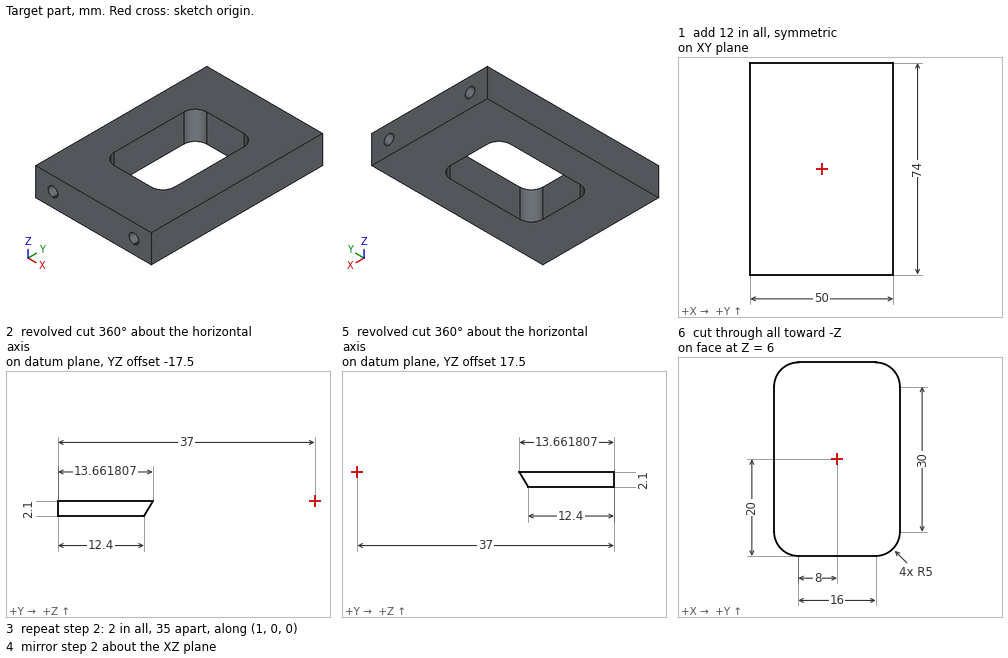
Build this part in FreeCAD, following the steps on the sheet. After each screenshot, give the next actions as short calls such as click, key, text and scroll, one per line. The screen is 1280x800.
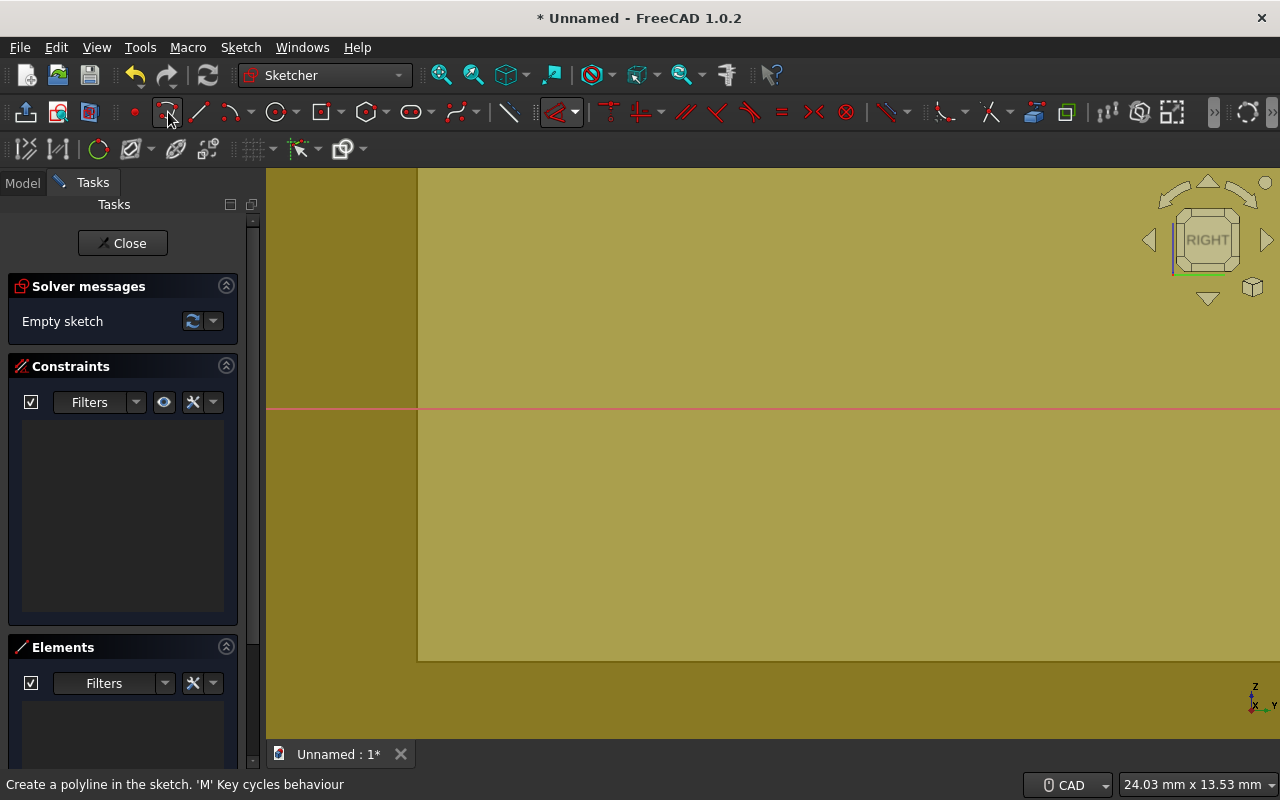
click(994, 409)
click(417, 418)
click(417, 497)
click(941, 497)
click(994, 409)
key(Escape)
key(Escape)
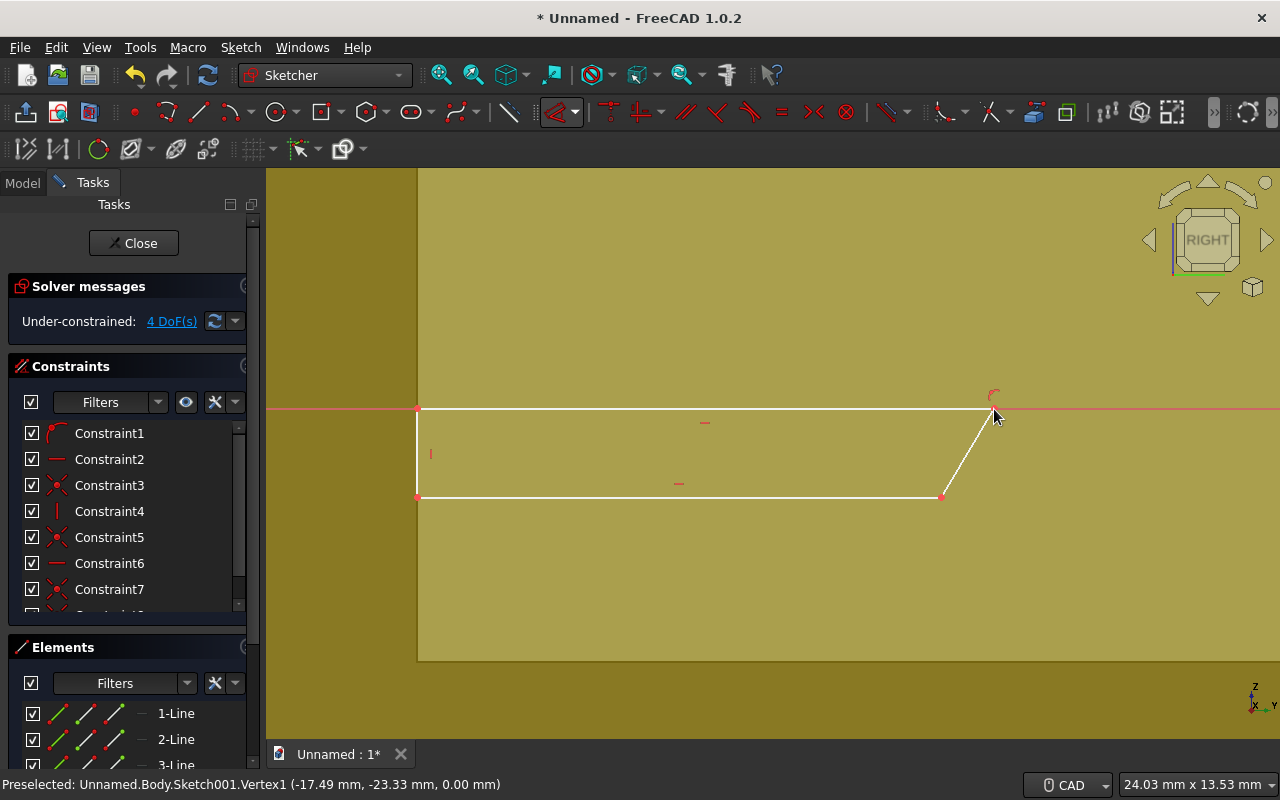
click(417, 435)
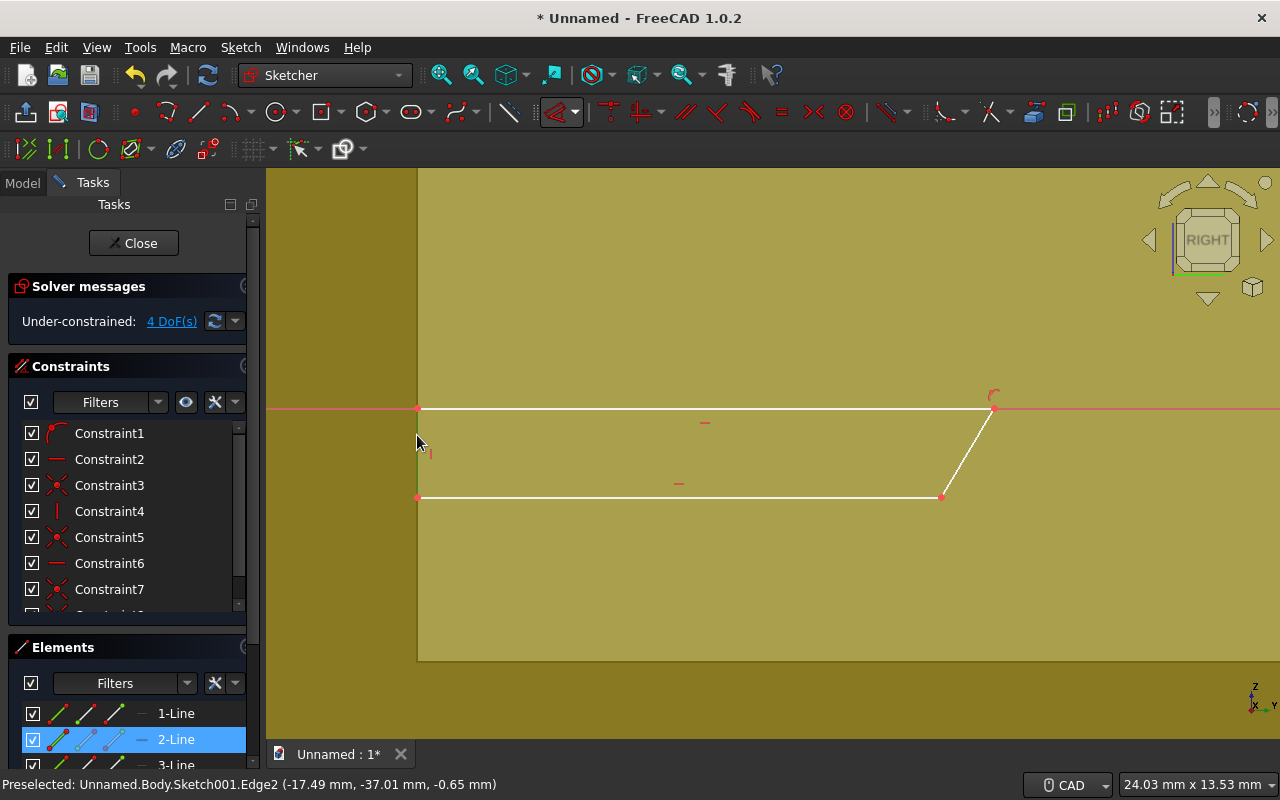
click(578, 112)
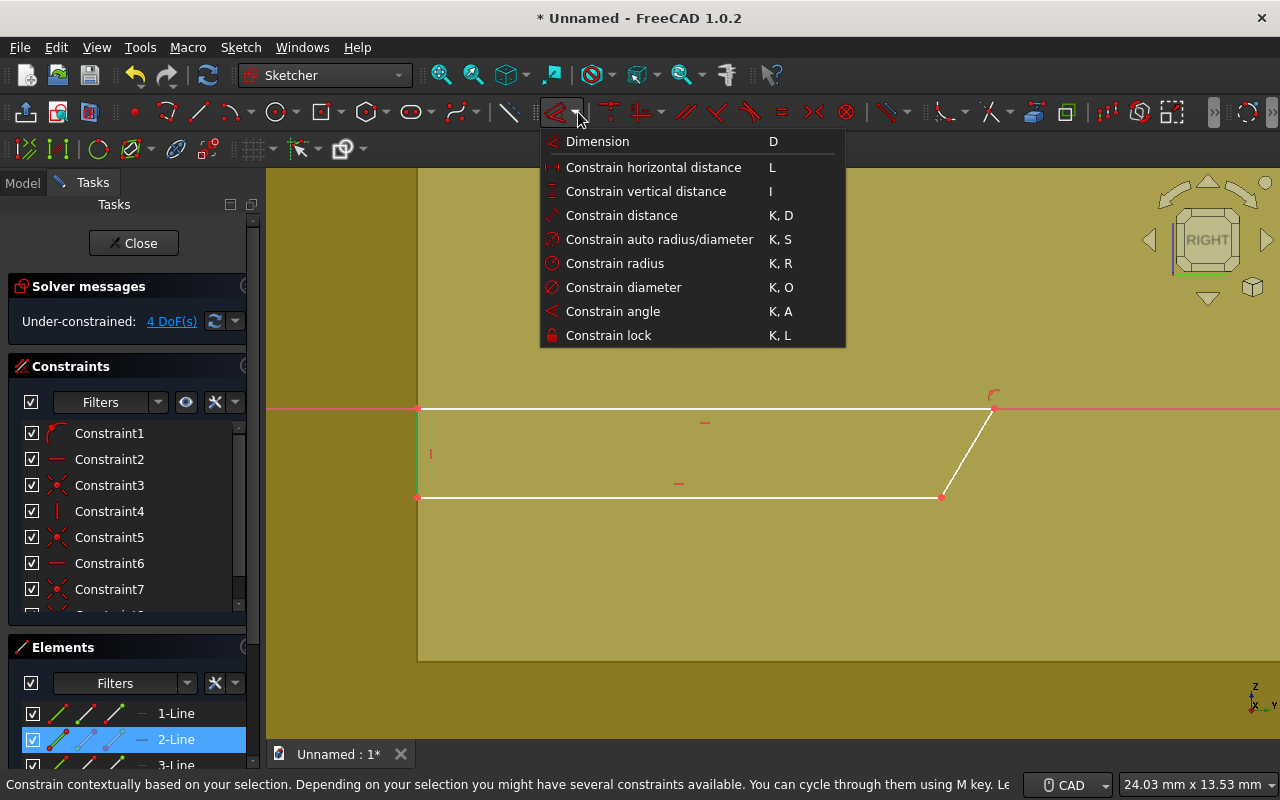
click(693, 191)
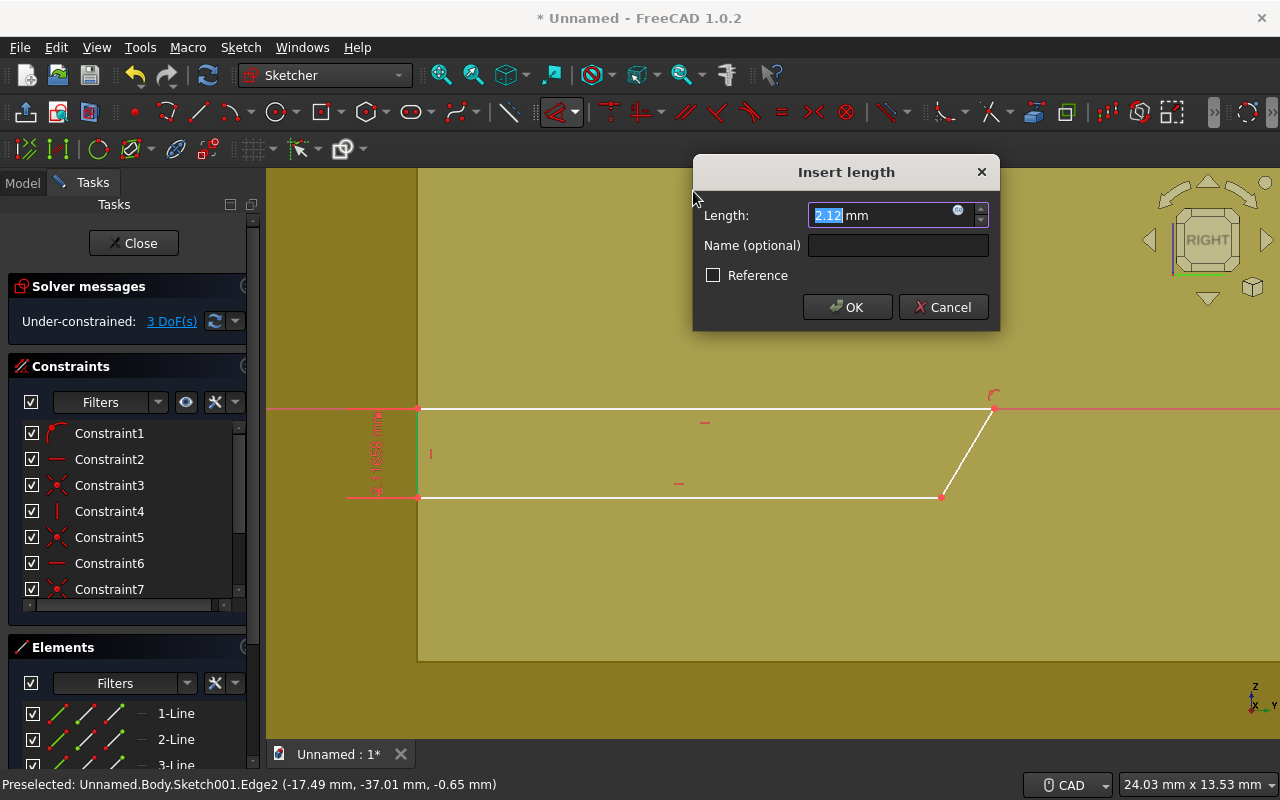
text(2.1)
key(Return)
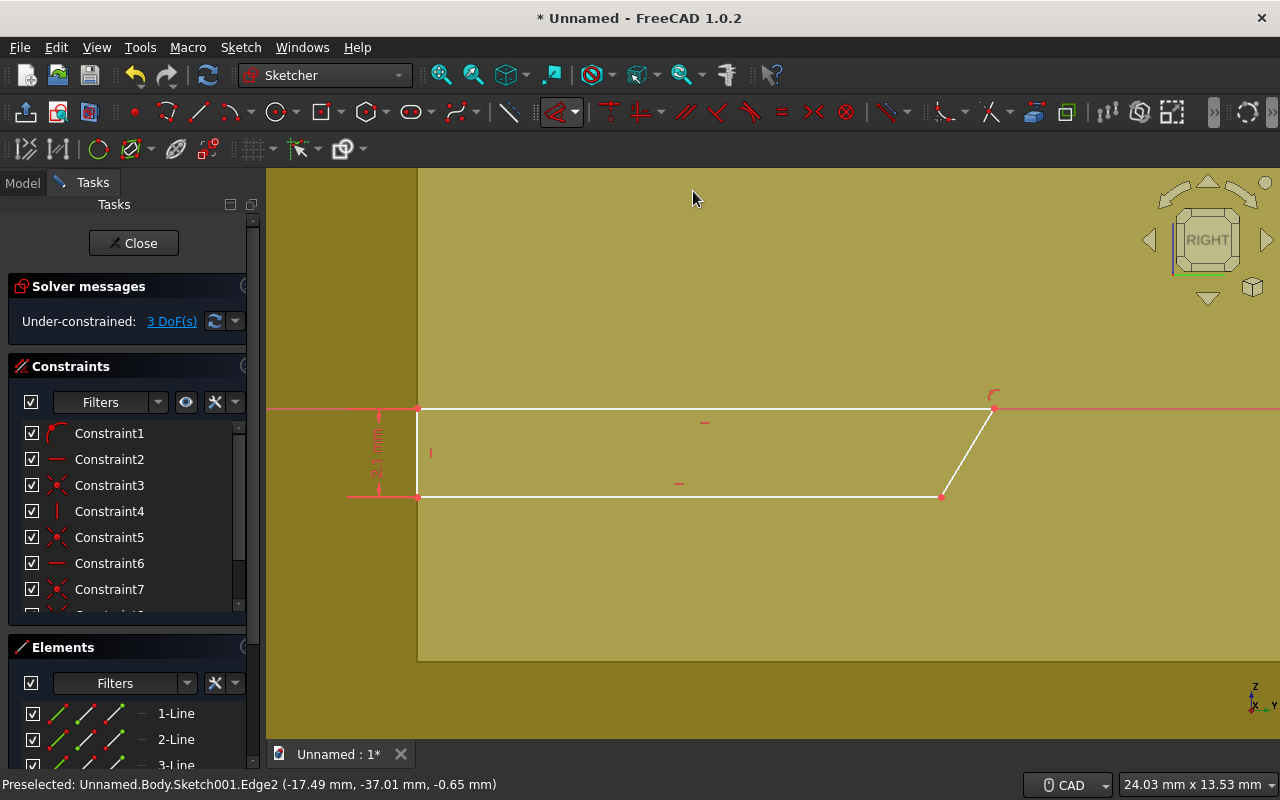
click(417, 409)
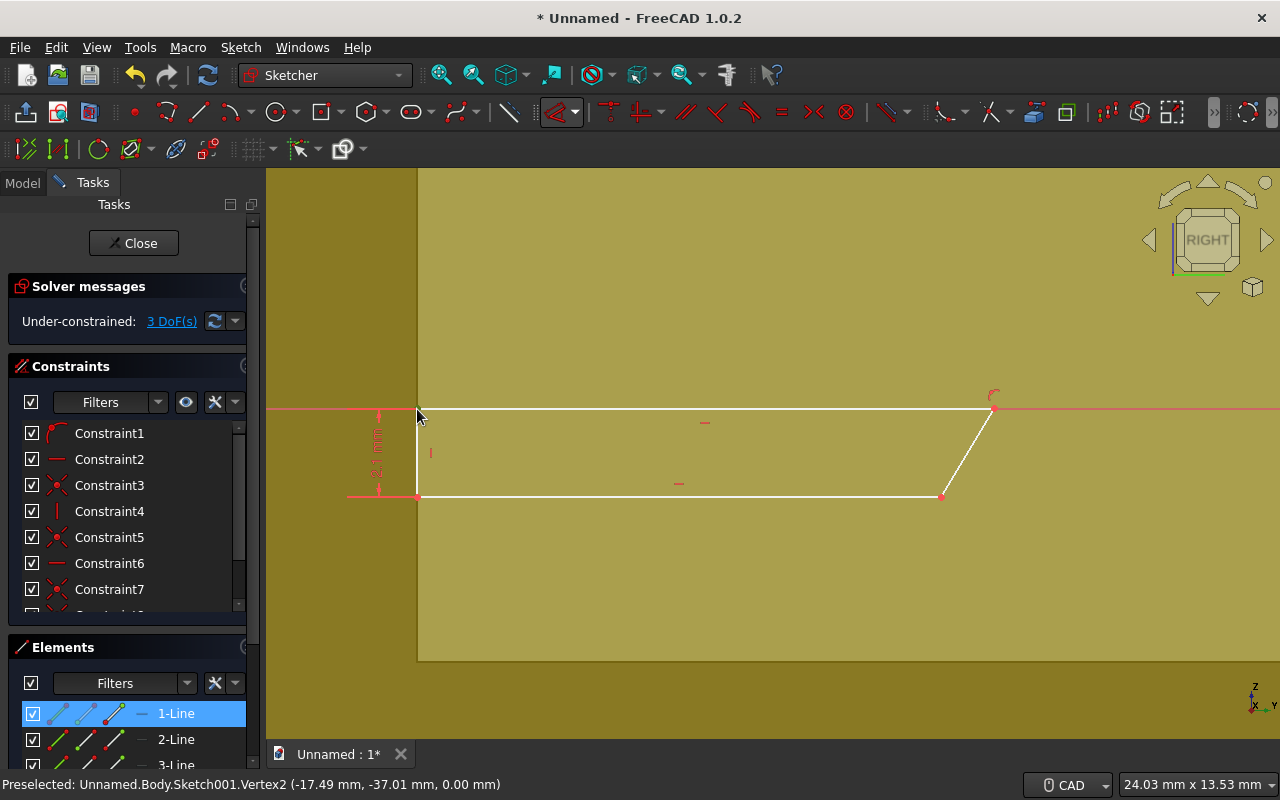
click(578, 112)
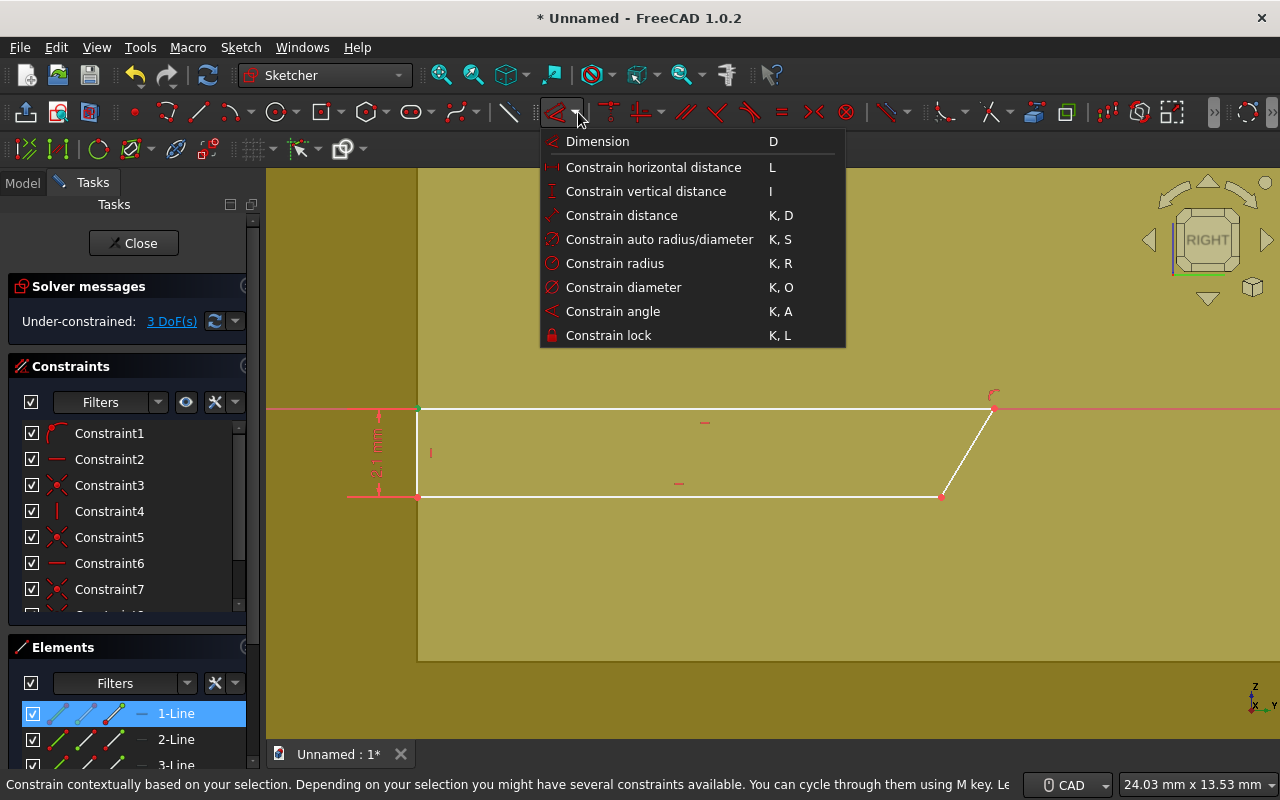
click(693, 167)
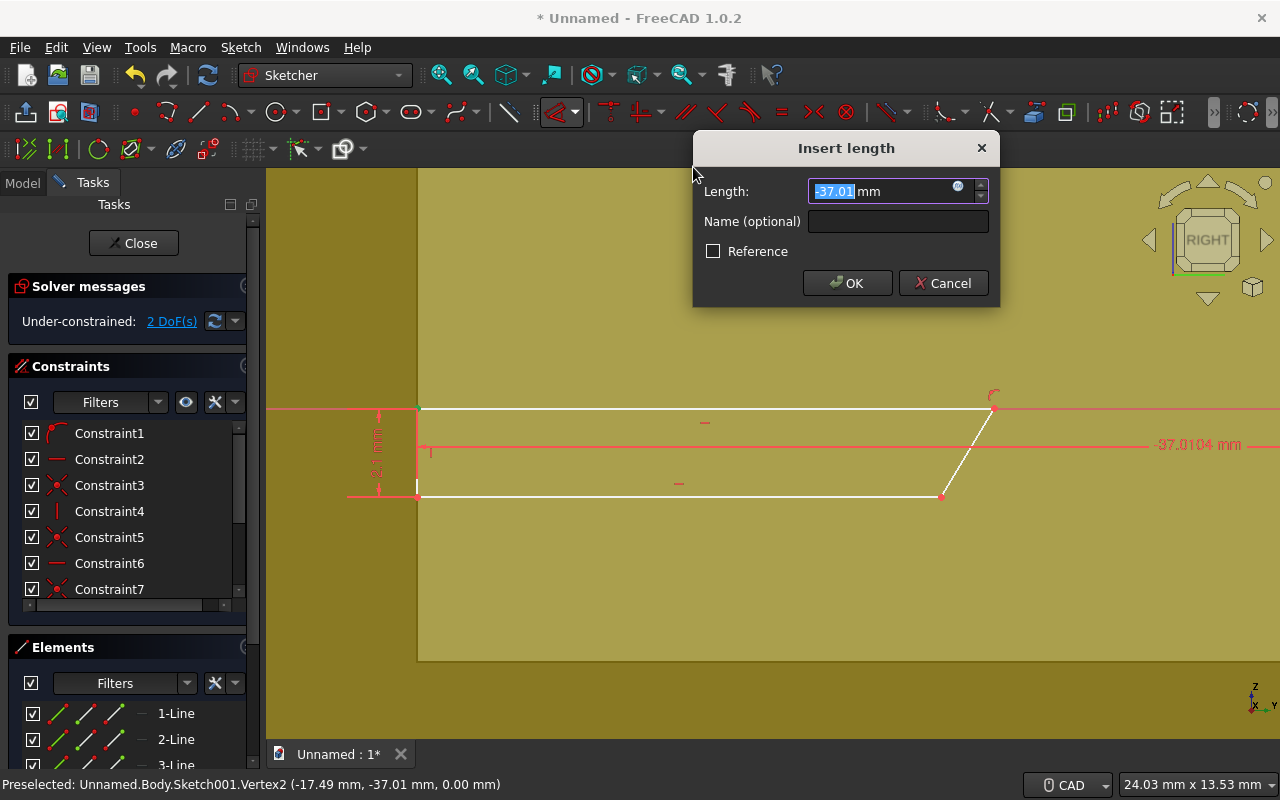
text(-37)
key(Return)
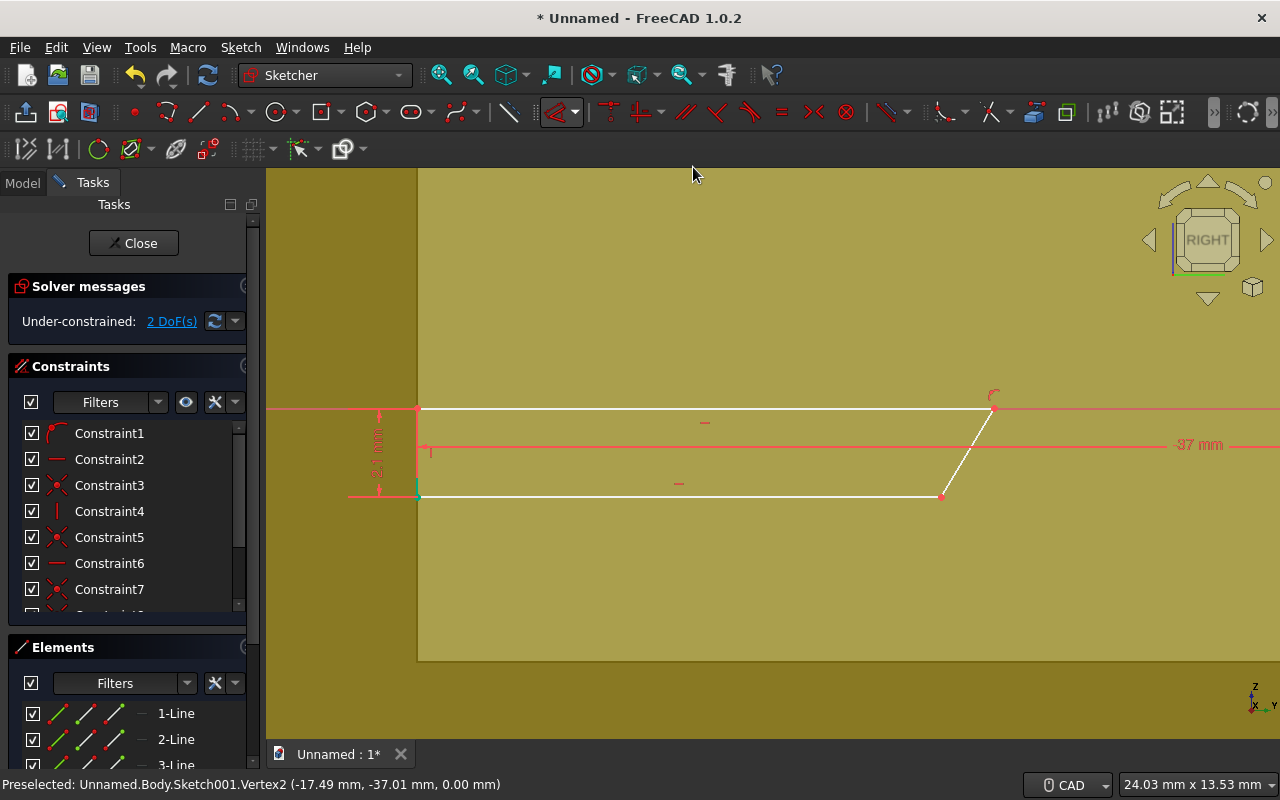
click(575, 497)